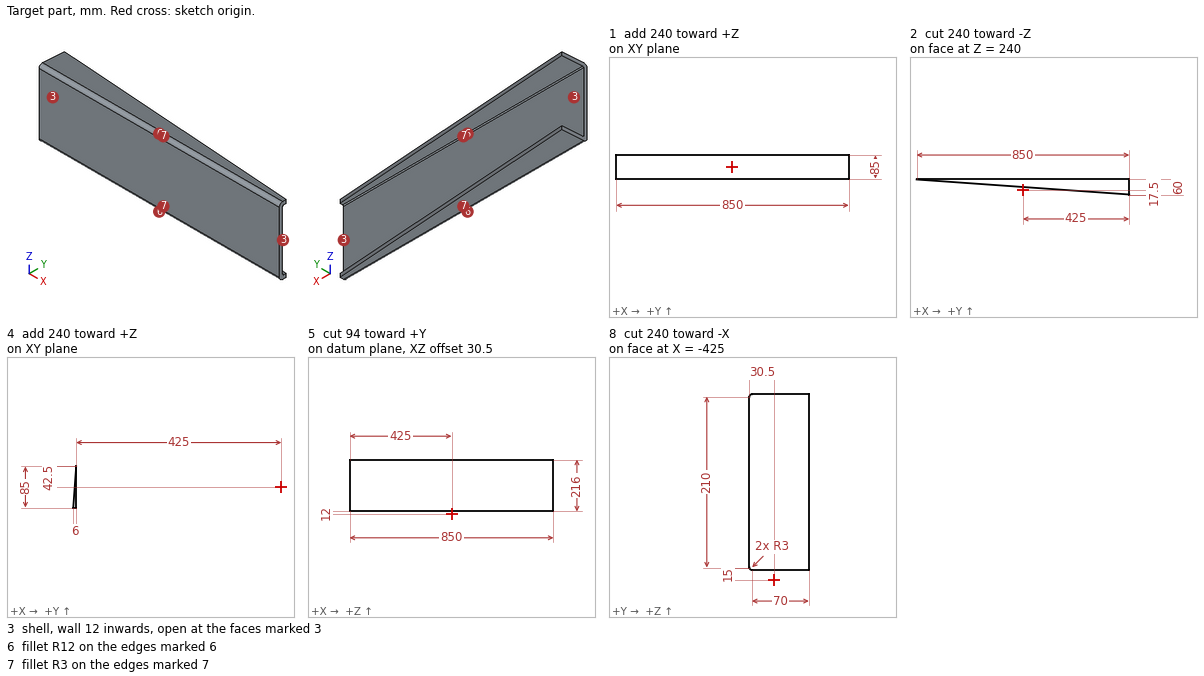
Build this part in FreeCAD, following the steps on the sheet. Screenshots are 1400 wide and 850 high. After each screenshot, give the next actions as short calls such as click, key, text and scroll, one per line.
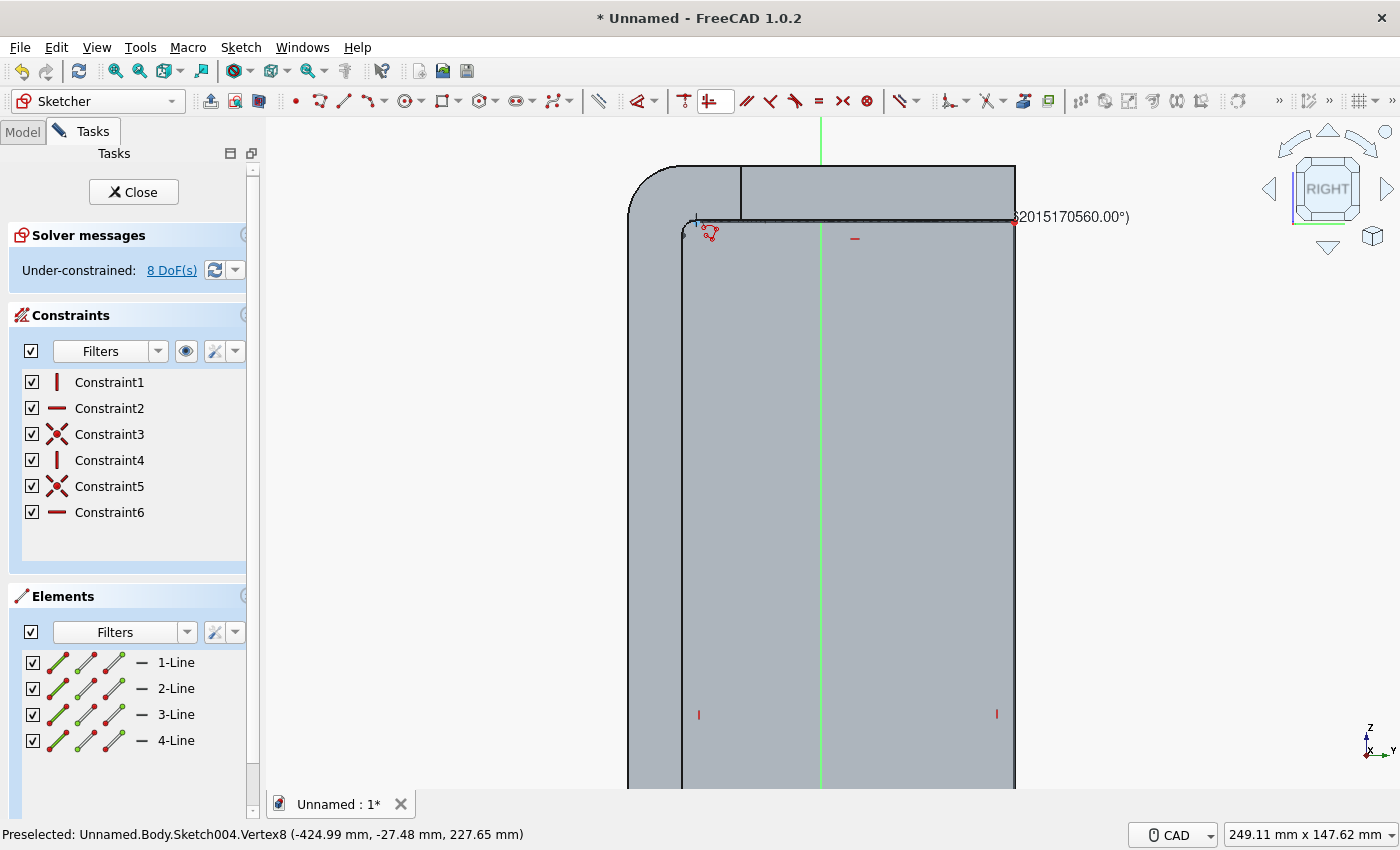
key(g)
key(3)
key(a)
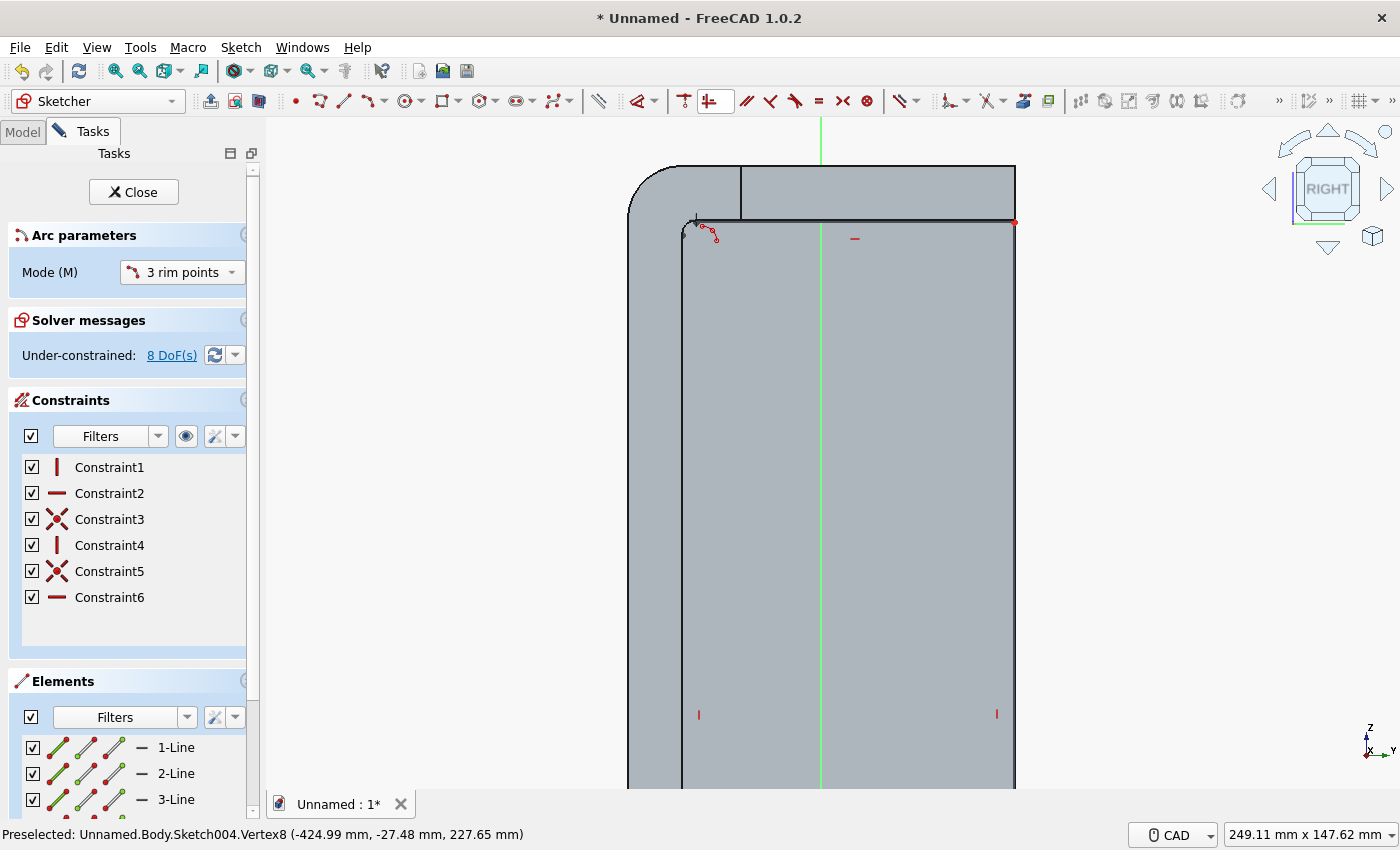
scroll(696, 219, down, 4)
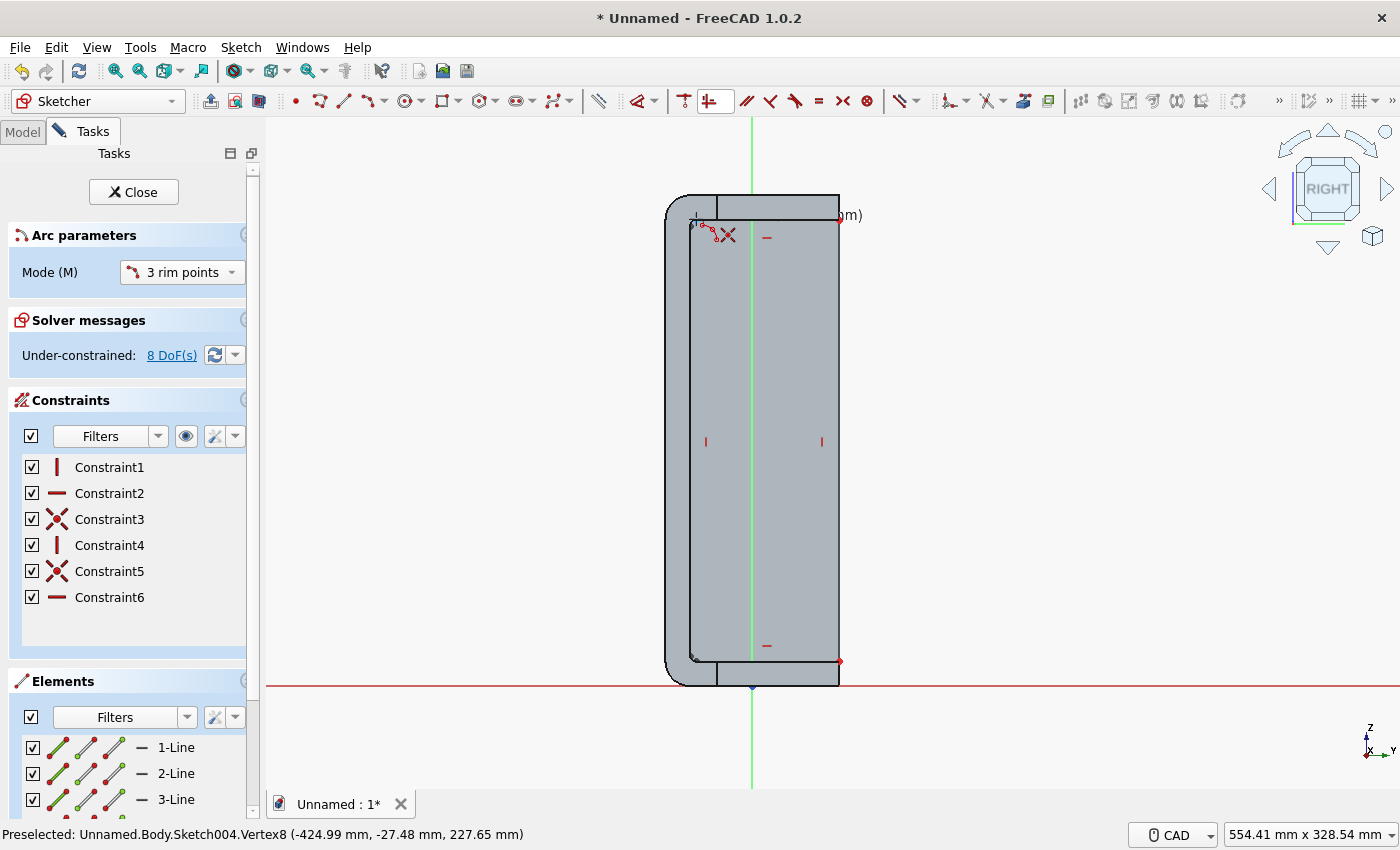
scroll(690, 655, up, 4)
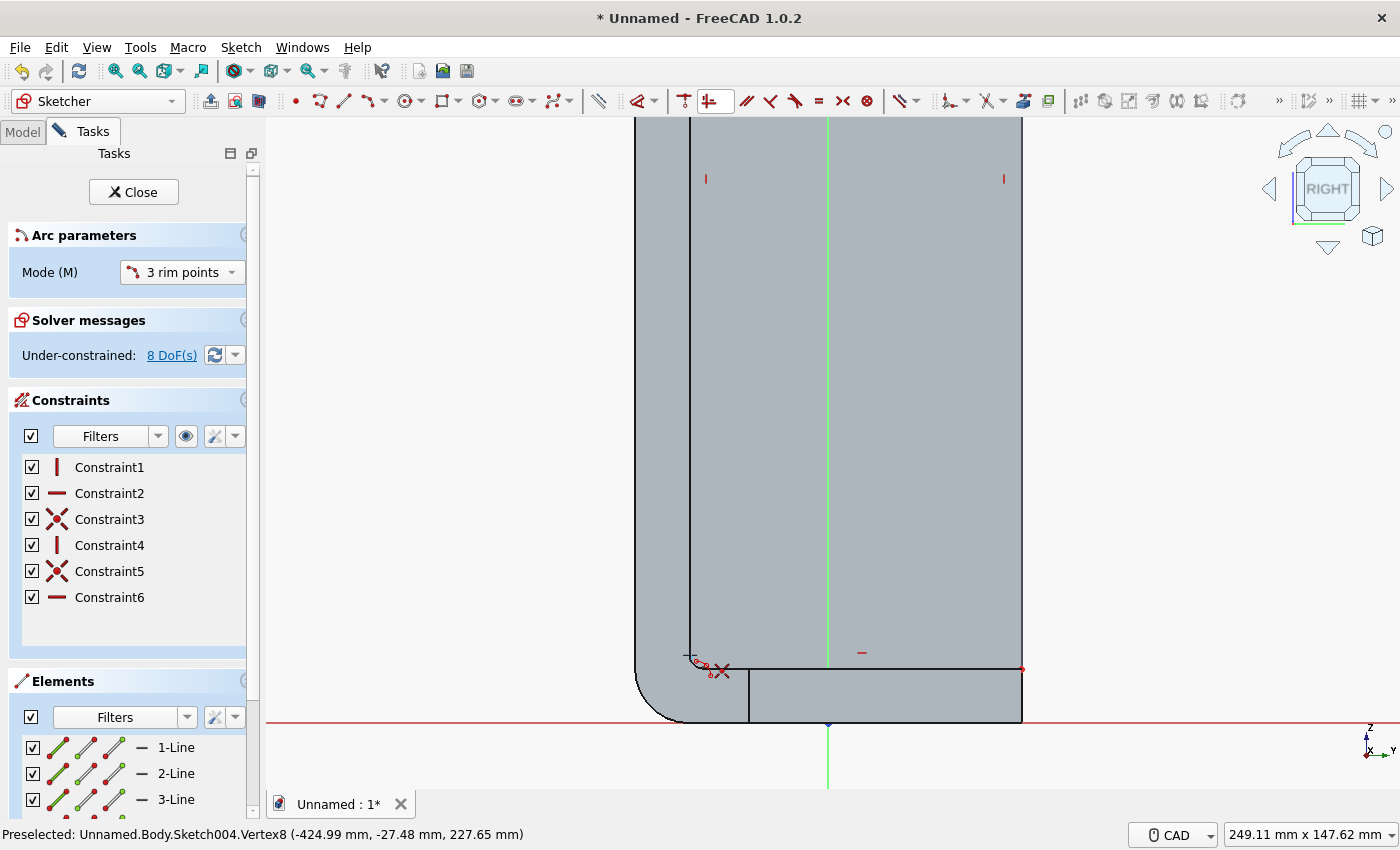
click(690, 657)
click(704, 670)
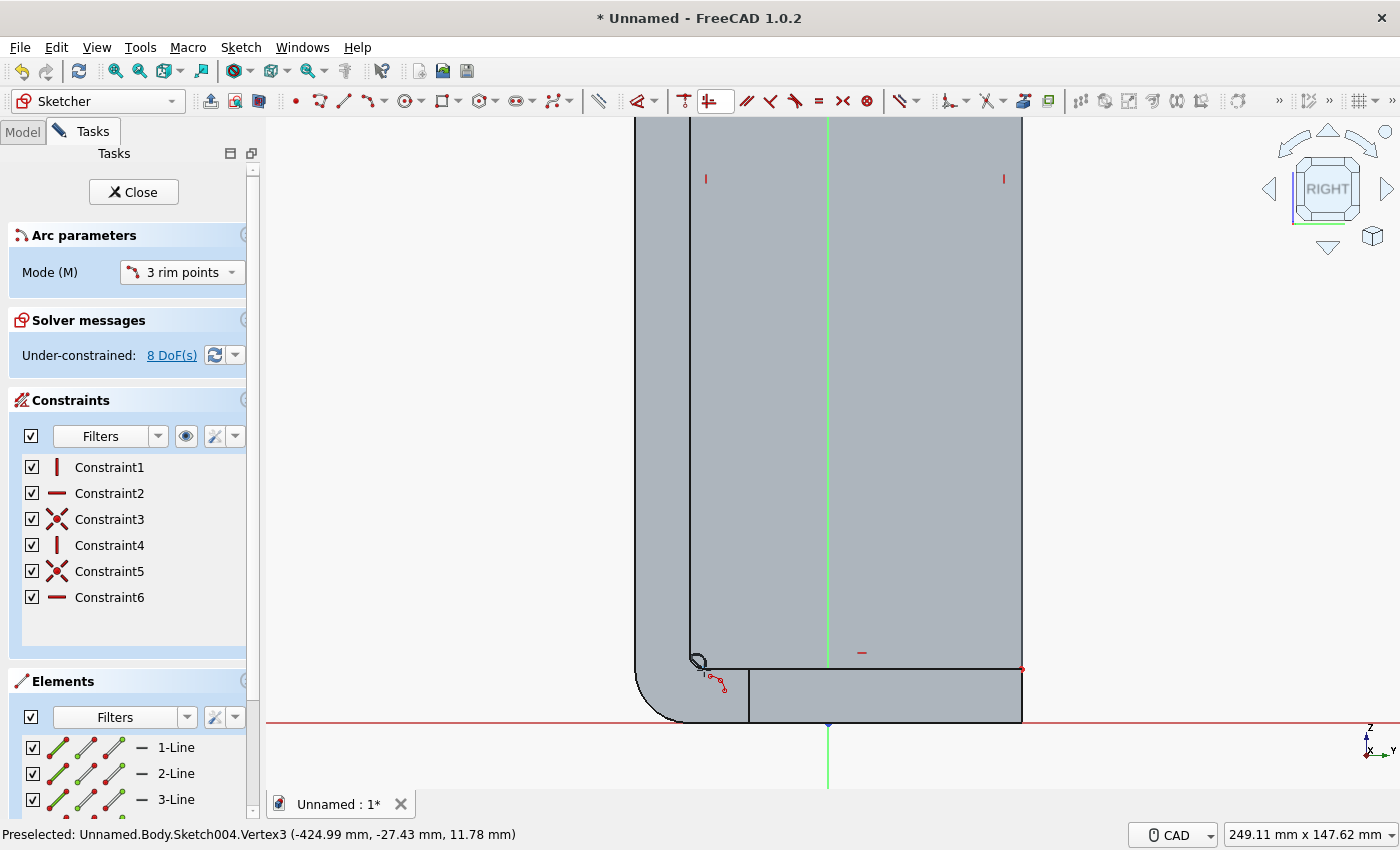
scroll(694, 665, up, 7)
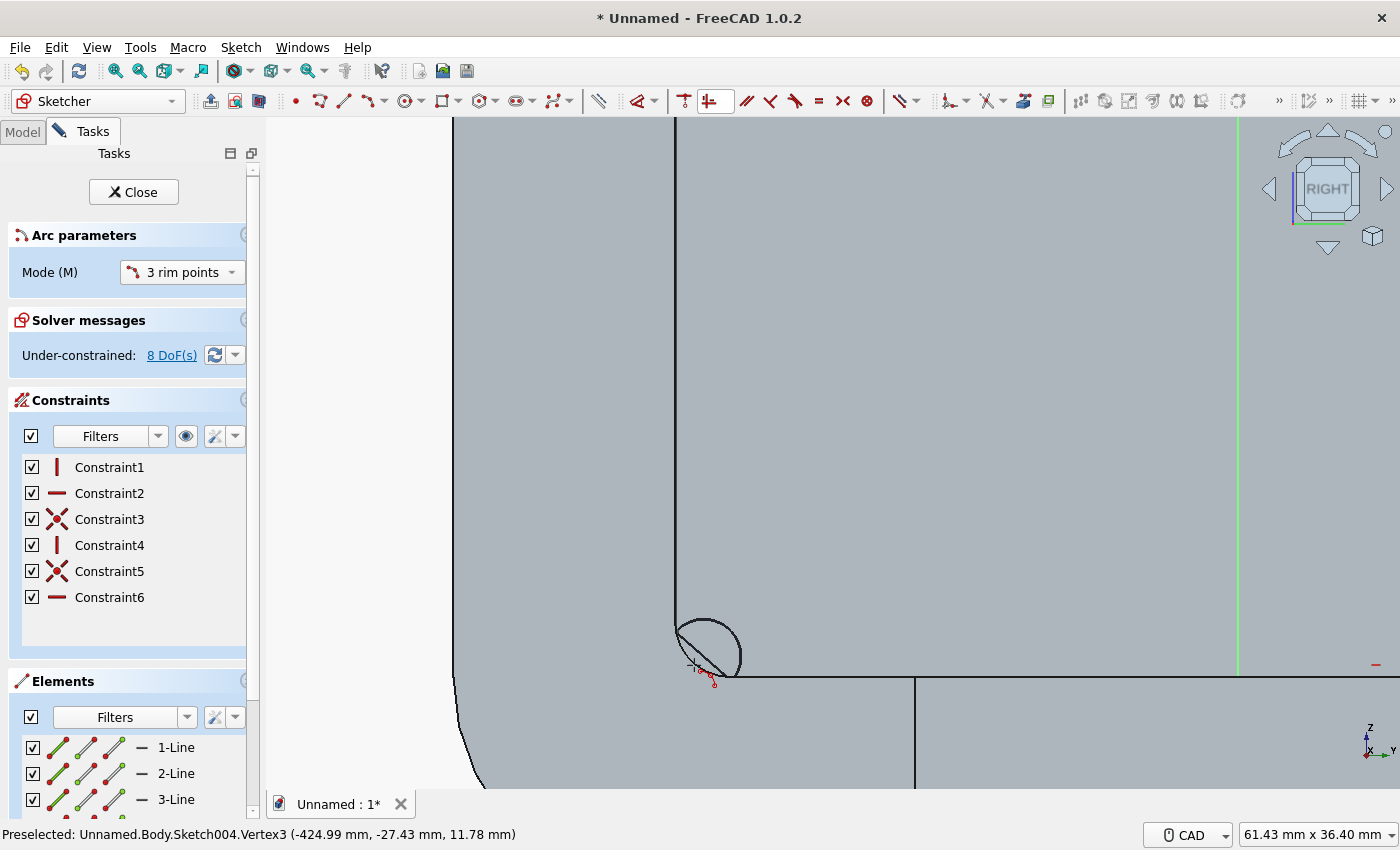
click(691, 661)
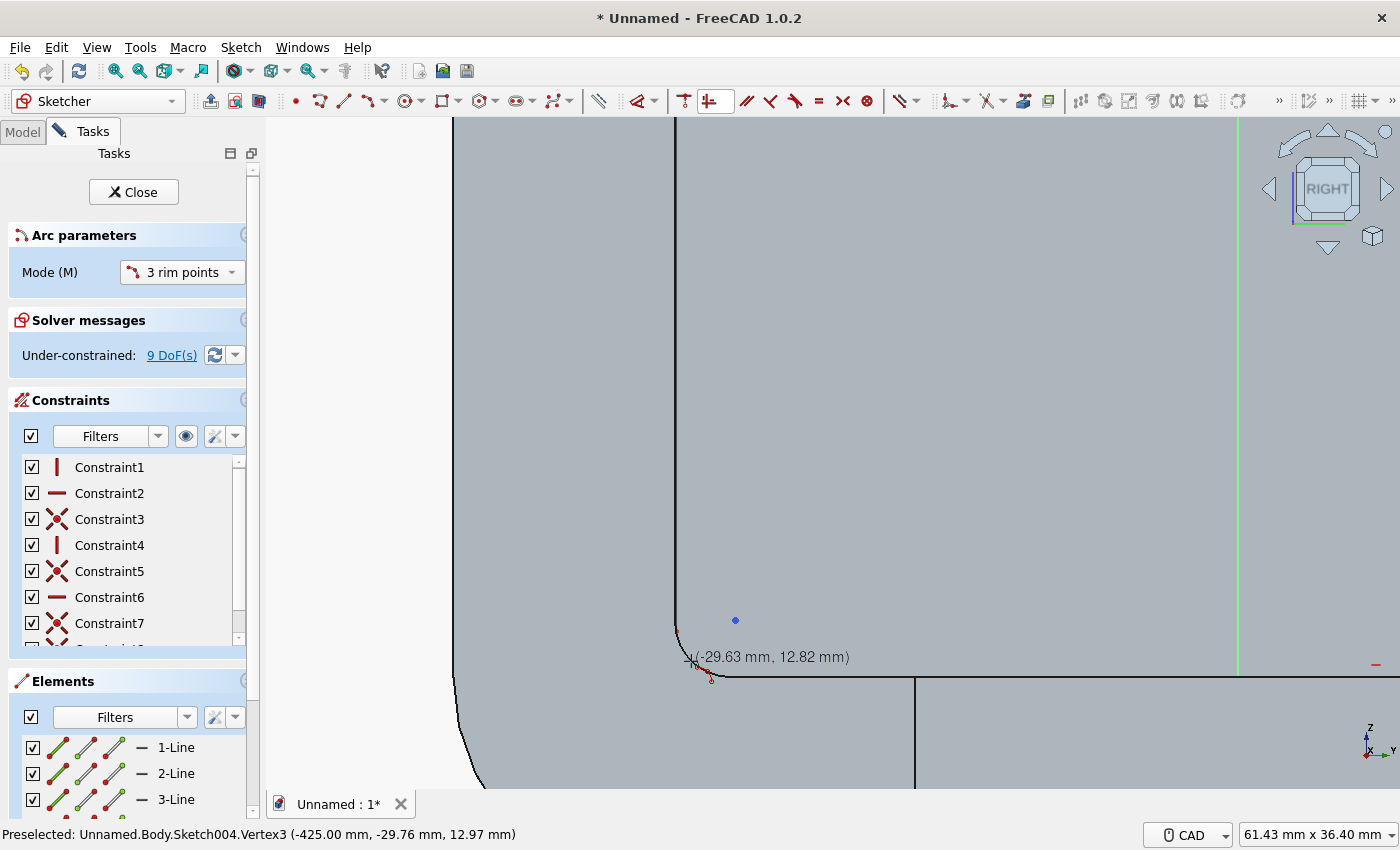
scroll(692, 660, down, 11)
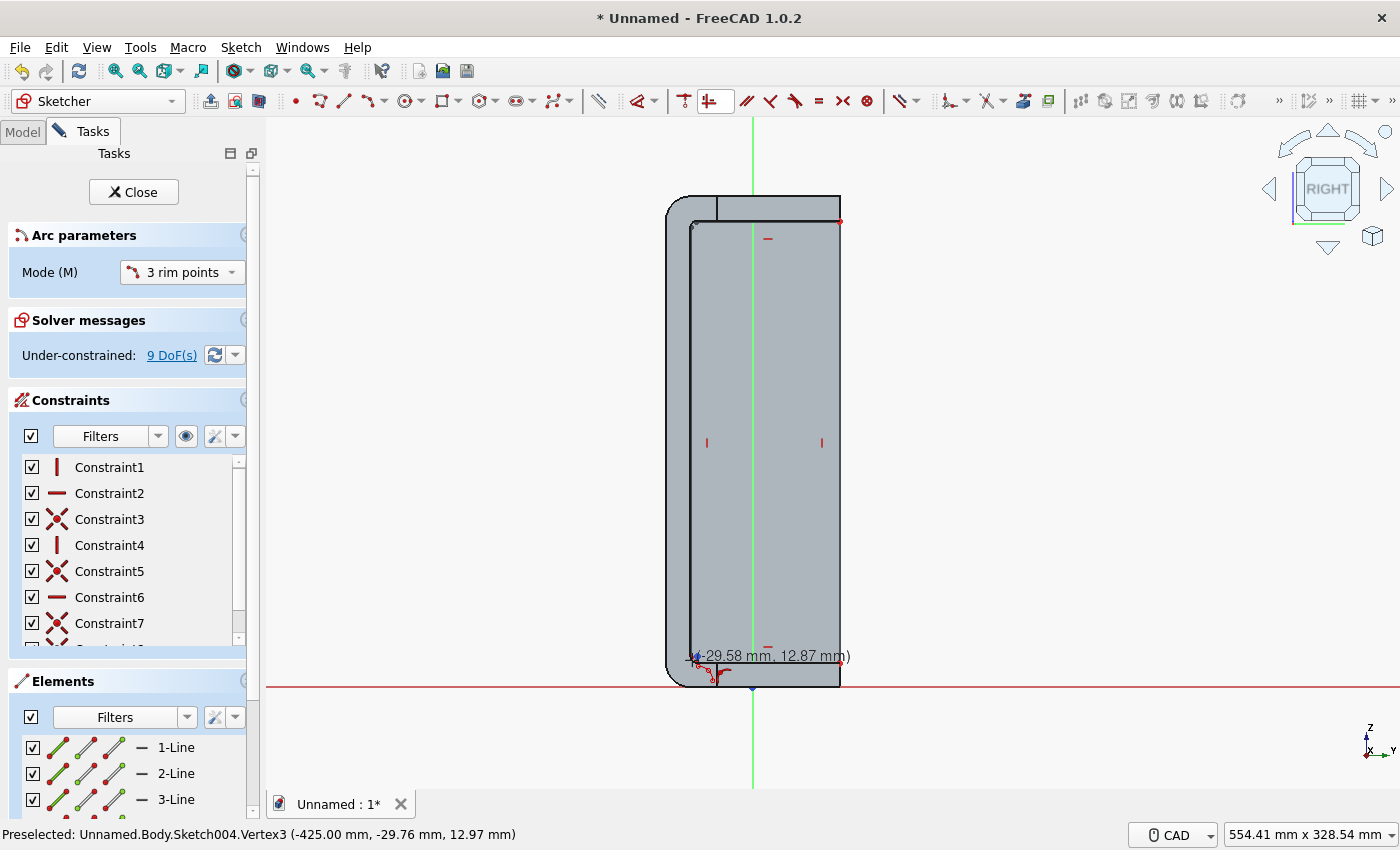
scroll(697, 221, up, 4)